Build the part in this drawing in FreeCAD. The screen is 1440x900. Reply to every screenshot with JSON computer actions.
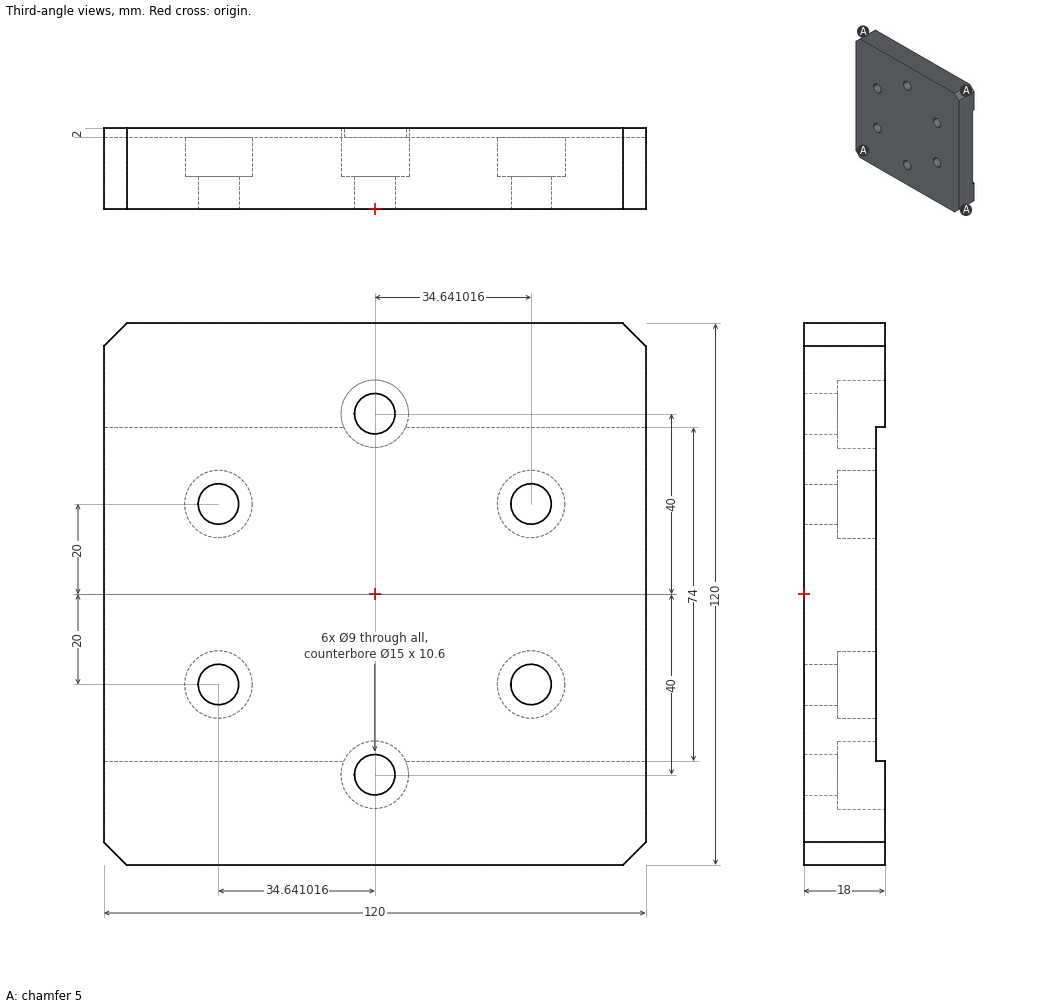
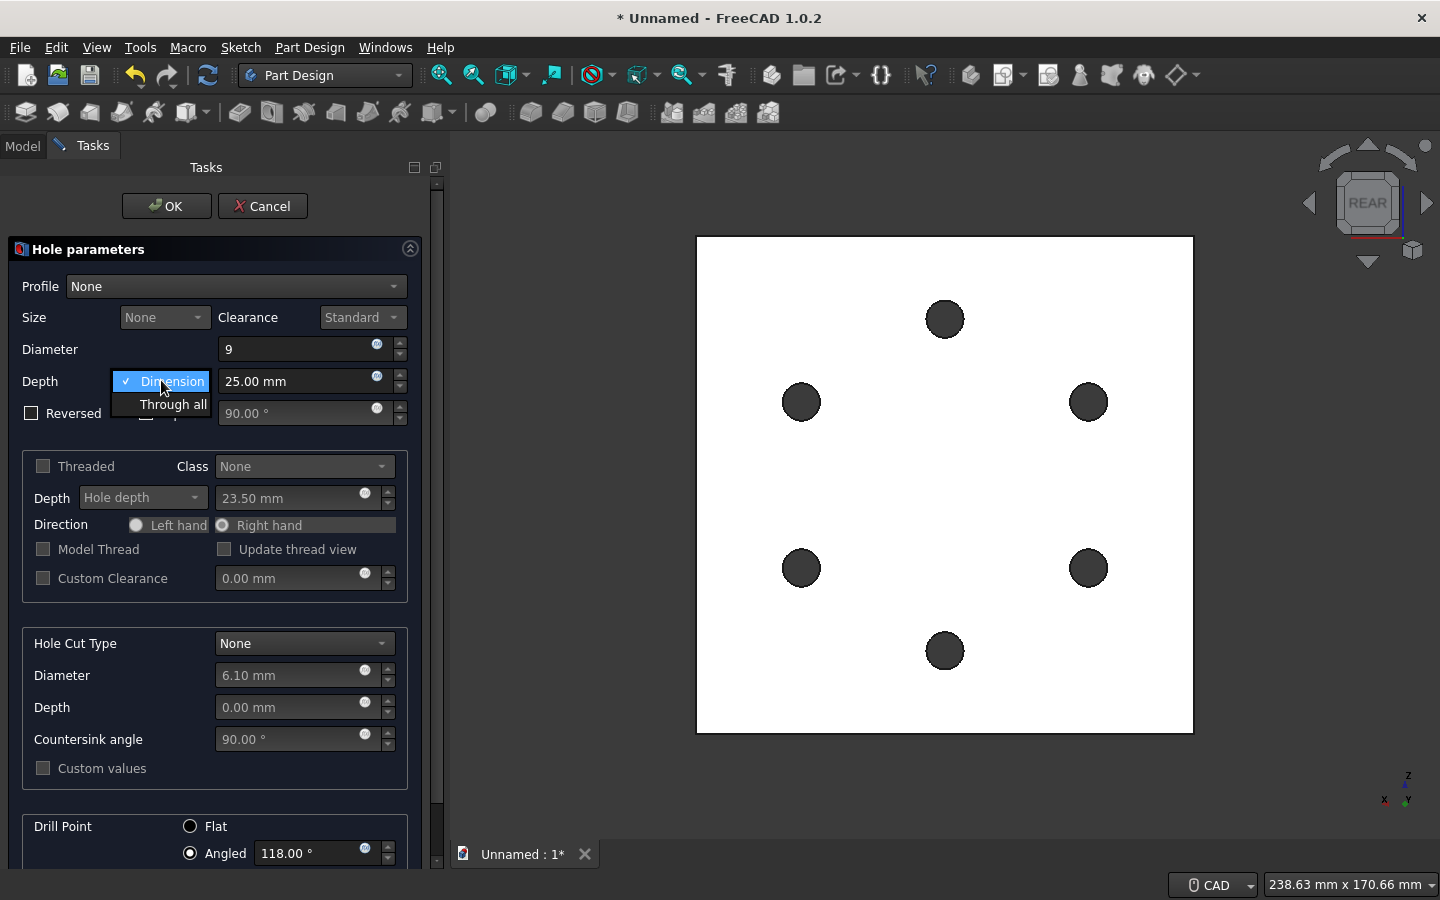
{"action": "left_click", "coordinate": [160, 404]}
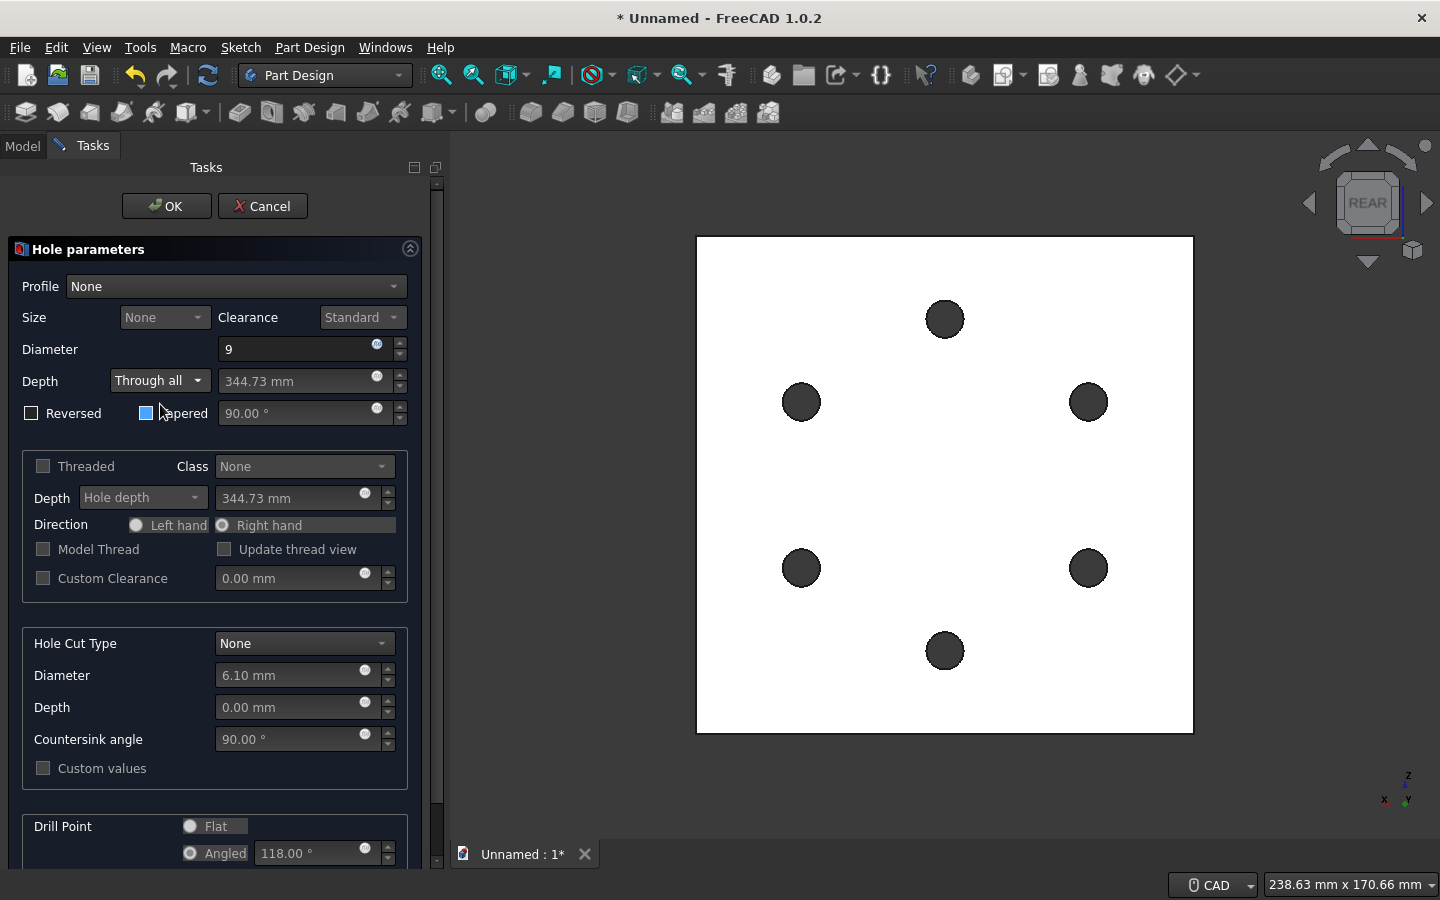
{"action": "left_click", "coordinate": [306, 644]}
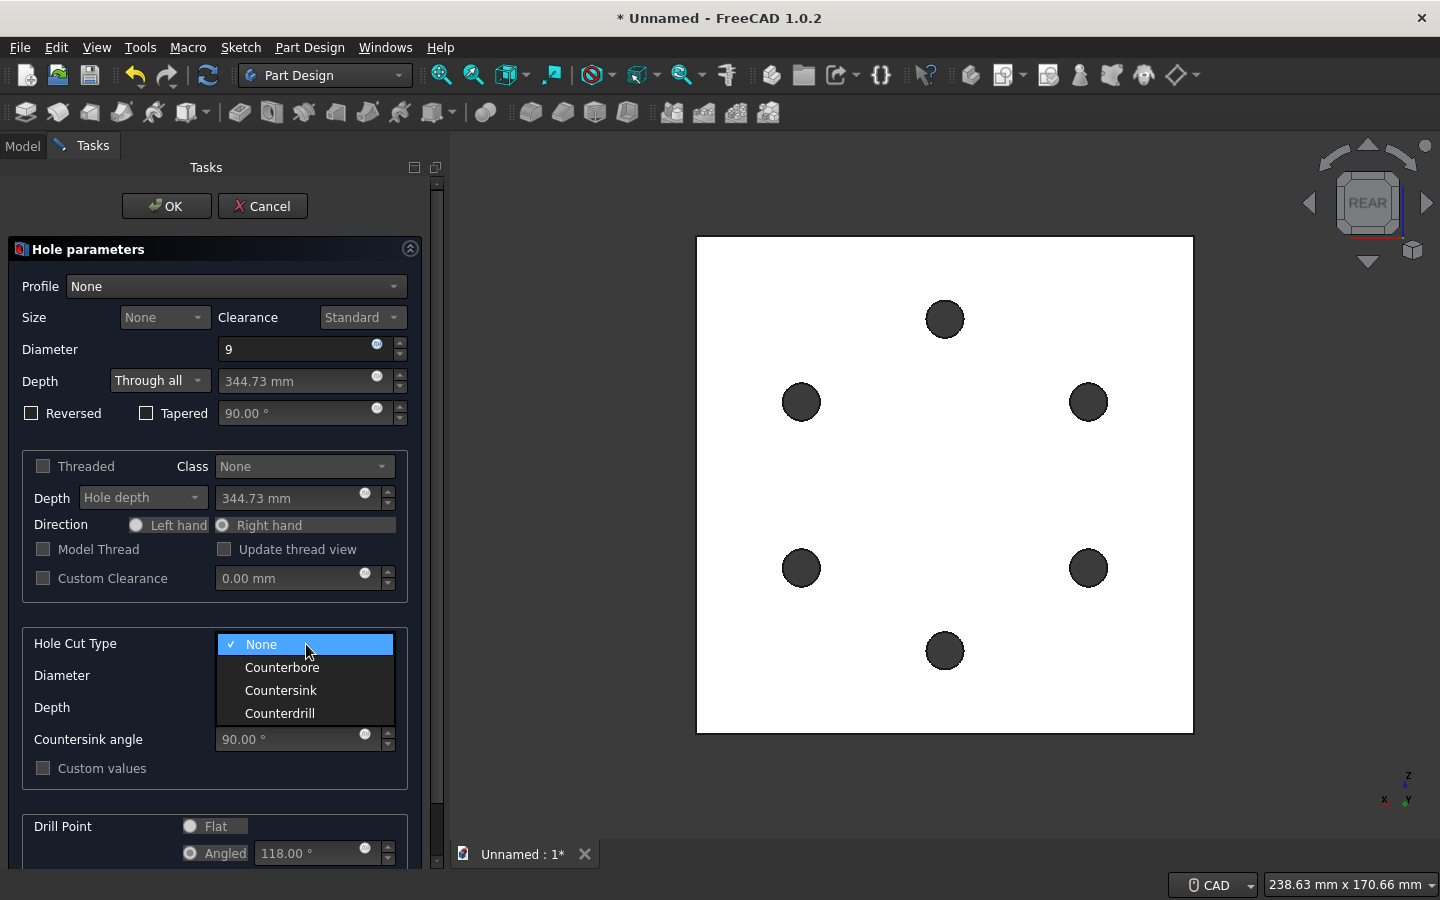
{"action": "left_click", "coordinate": [304, 668]}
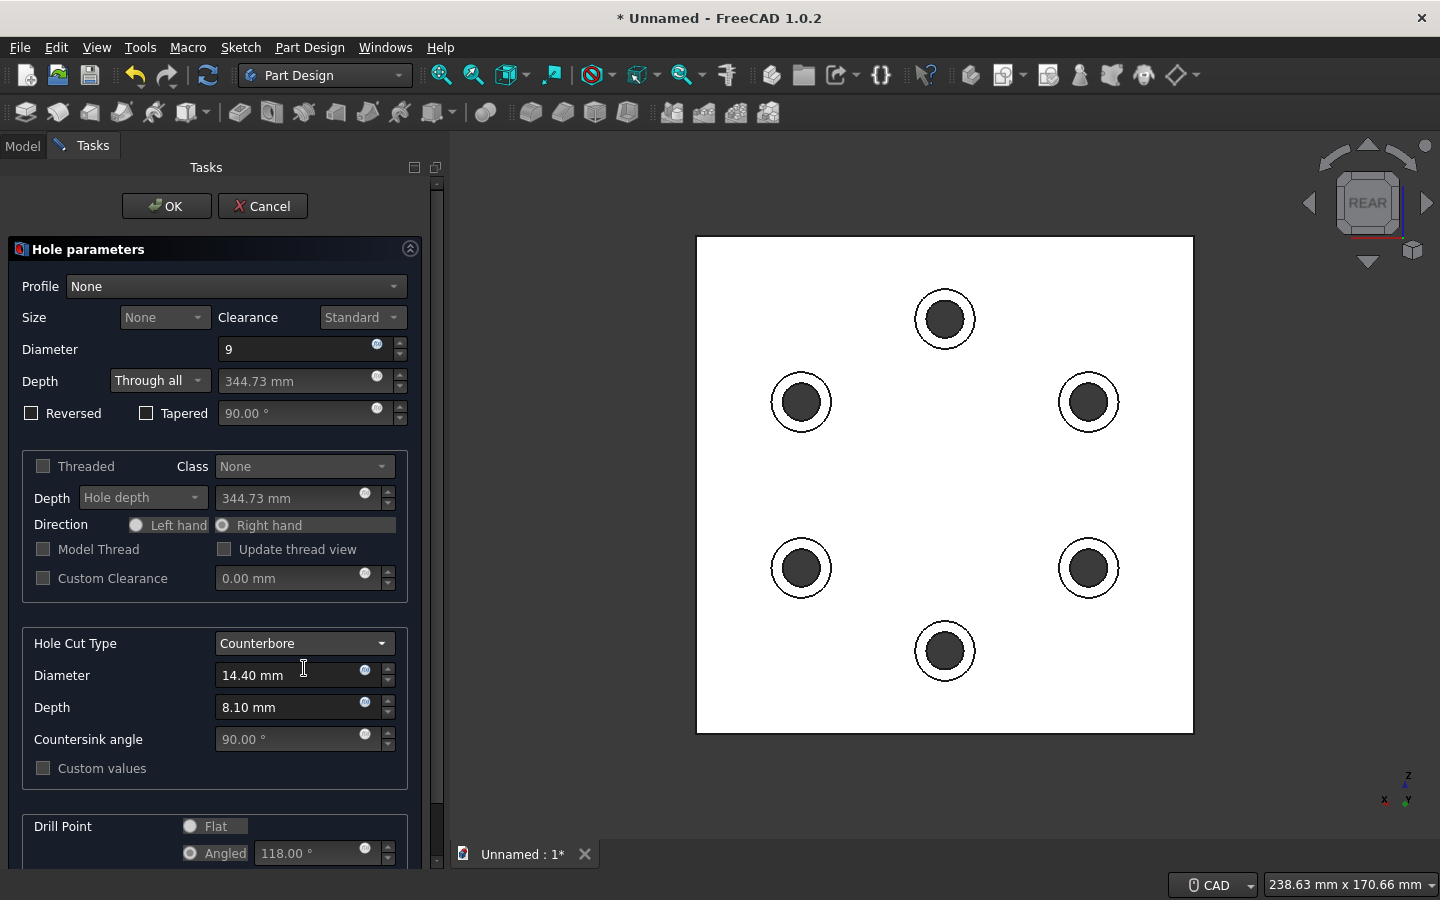
{"action": "triple_click", "coordinate": [298, 675]}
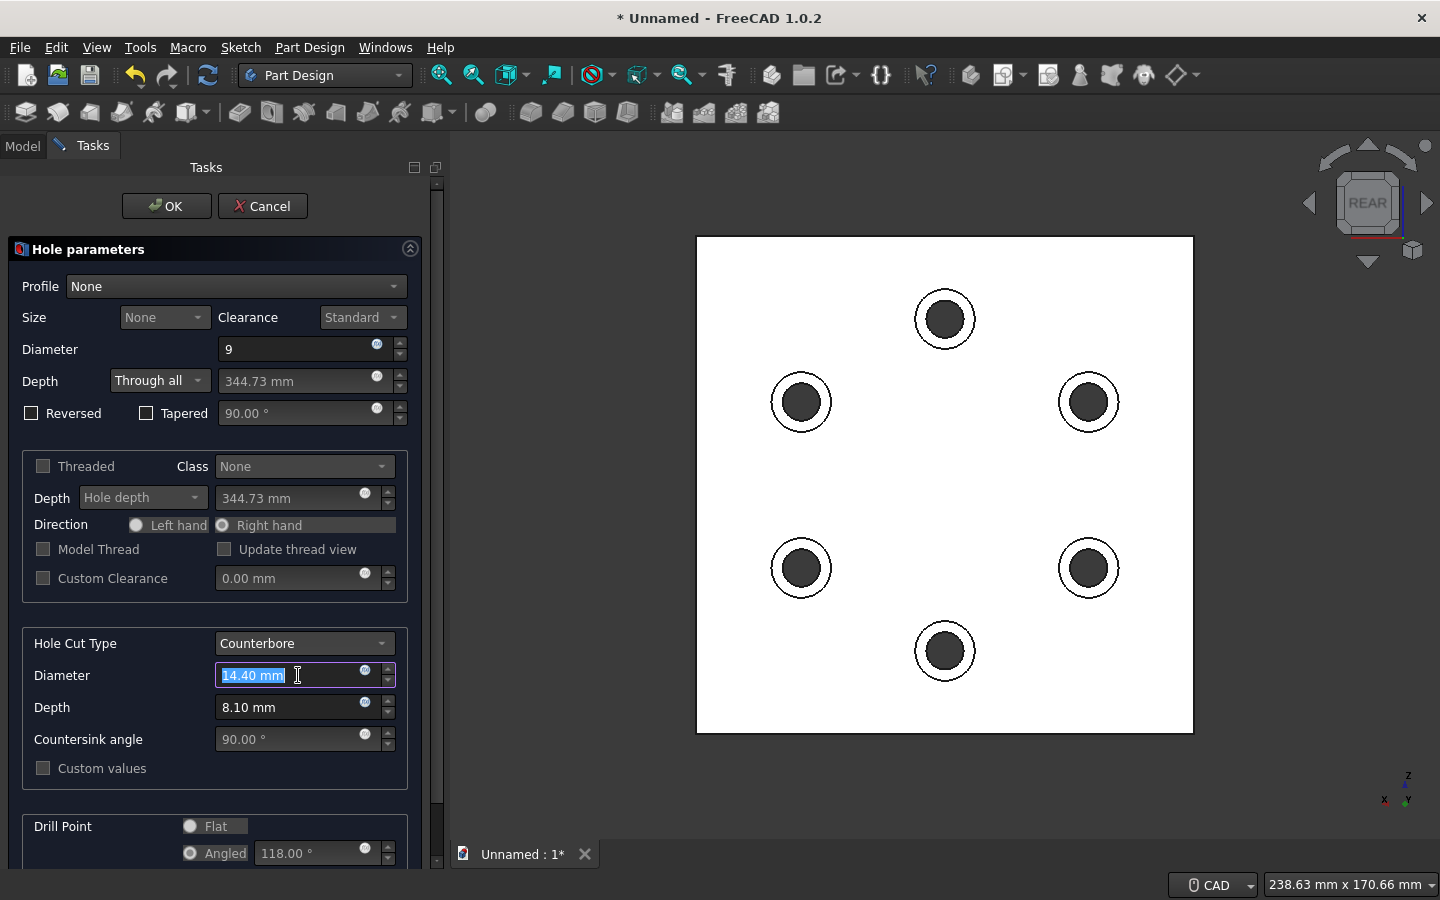
{"action": "type", "text": "15"}
{"action": "key", "text": "Tab"}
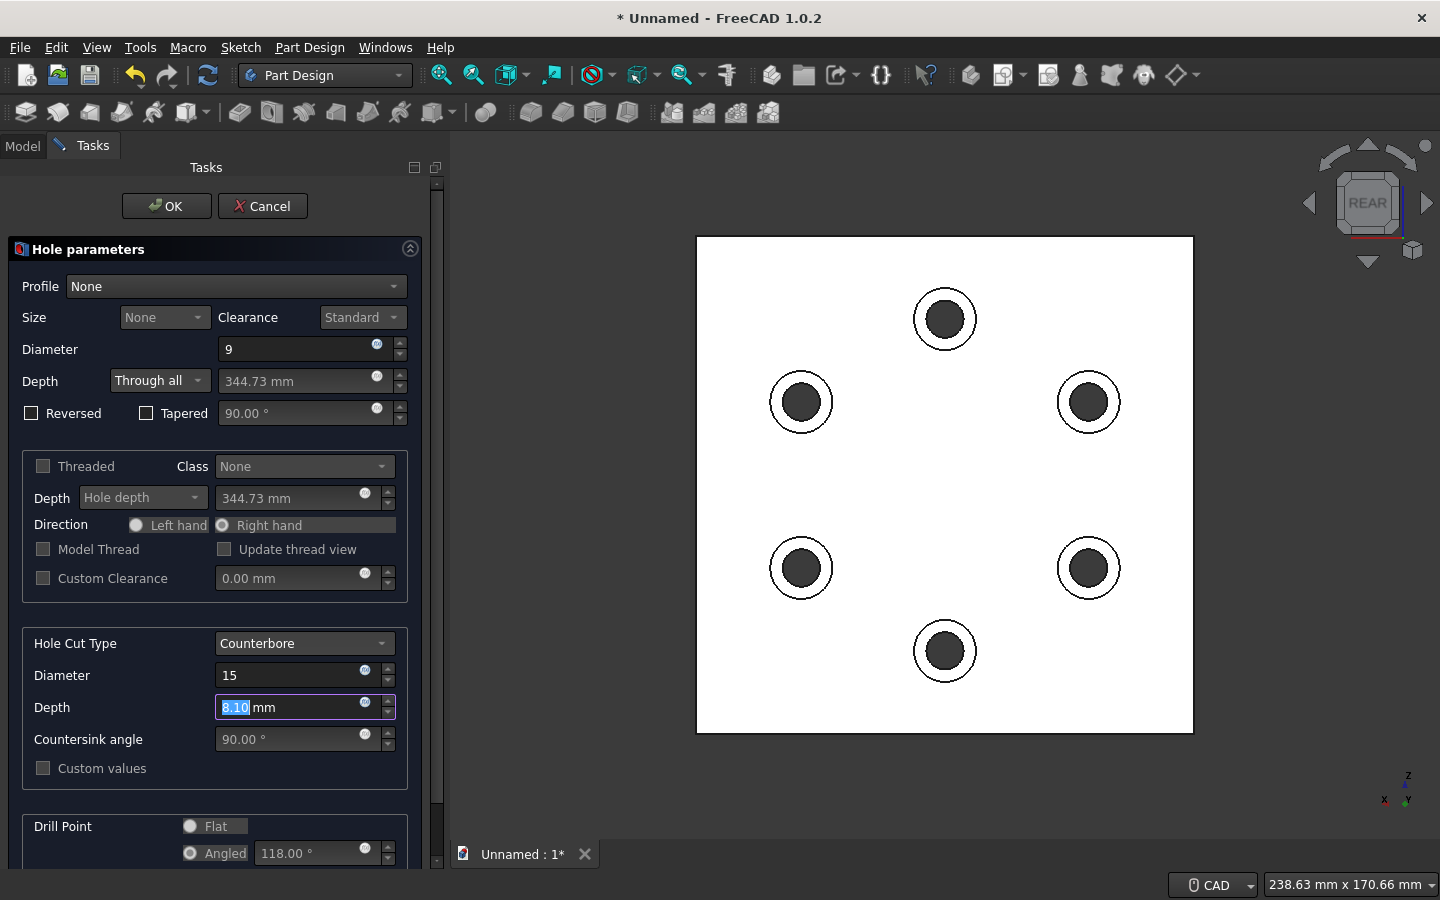
{"action": "type", "text": "10.6"}
{"action": "key", "text": "Tab"}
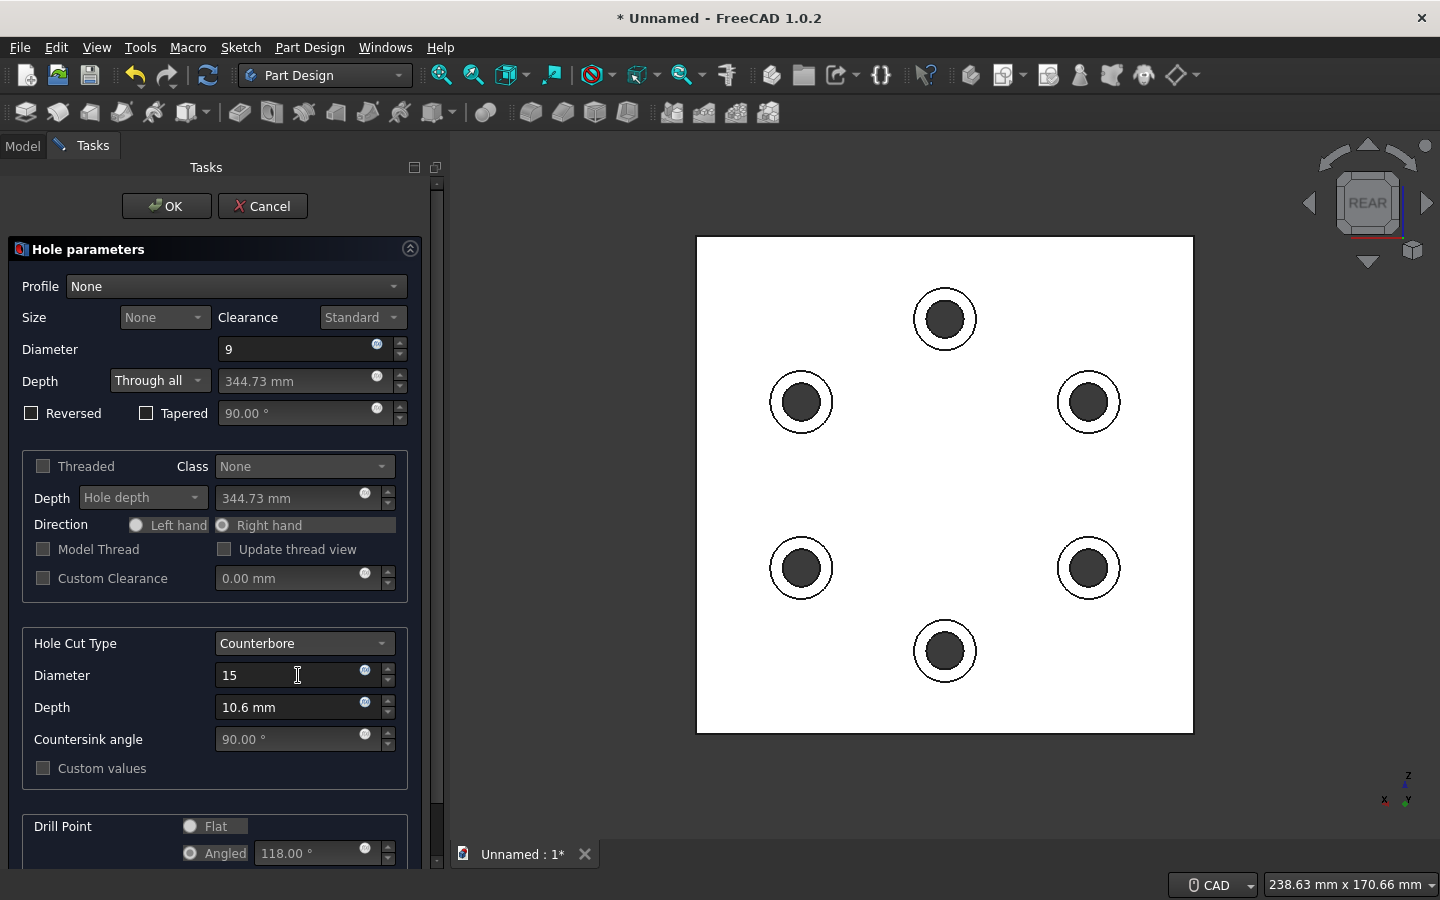
{"action": "left_click", "coordinate": [167, 206]}